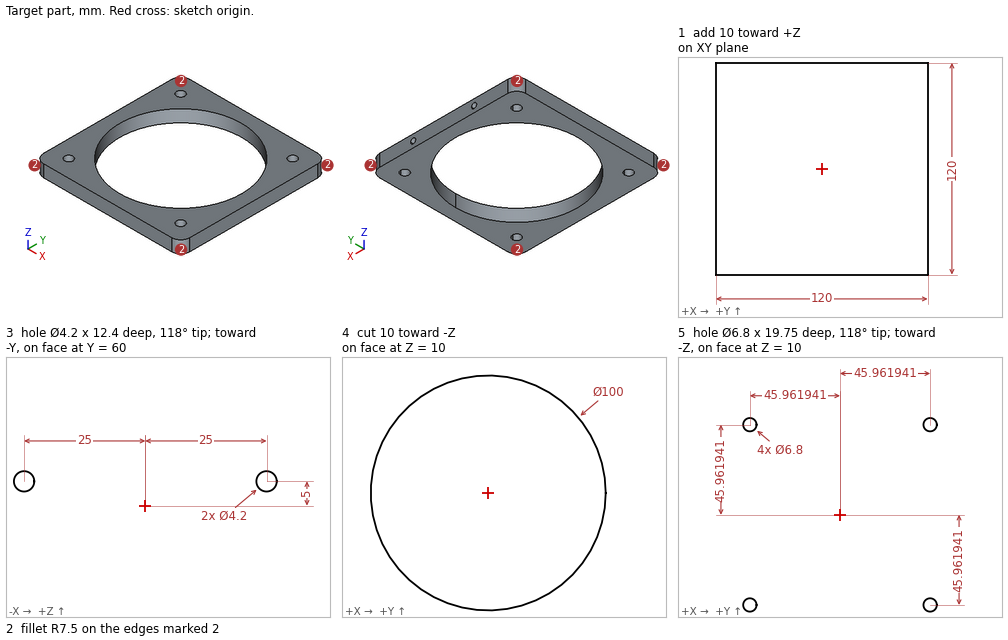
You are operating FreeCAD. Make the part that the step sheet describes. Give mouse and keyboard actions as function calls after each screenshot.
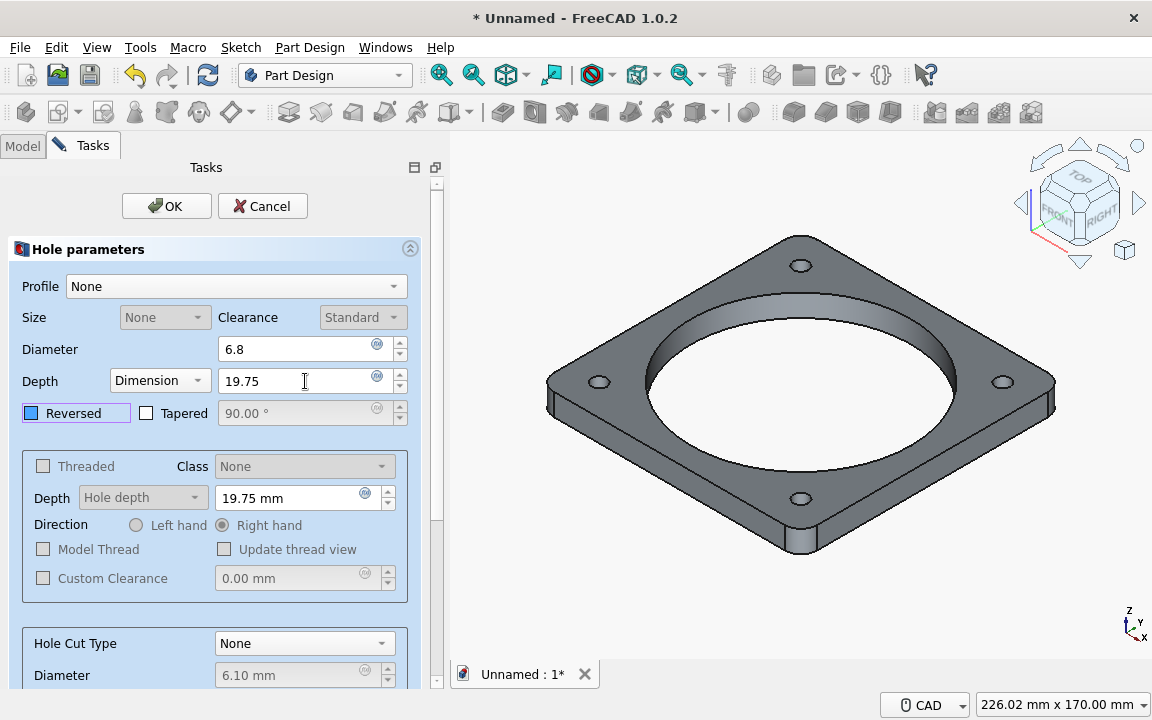
click(167, 206)